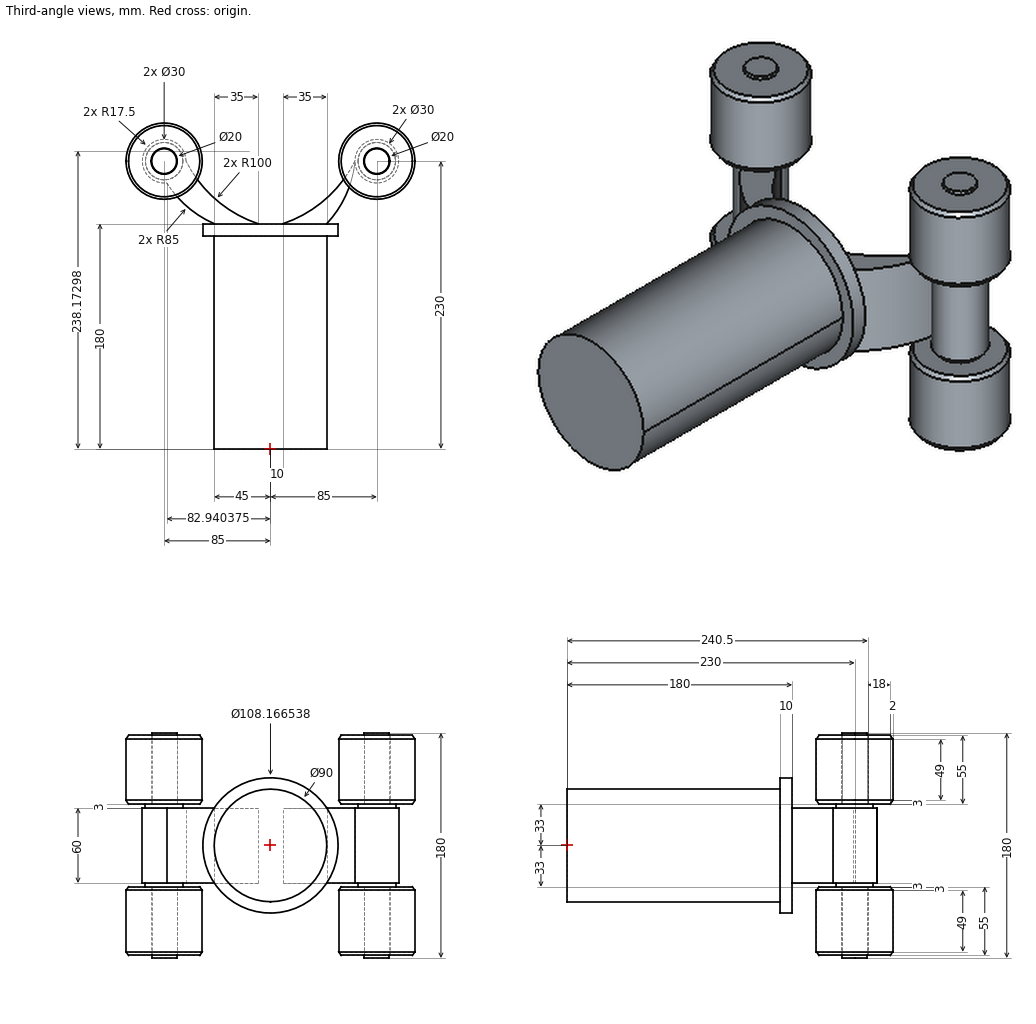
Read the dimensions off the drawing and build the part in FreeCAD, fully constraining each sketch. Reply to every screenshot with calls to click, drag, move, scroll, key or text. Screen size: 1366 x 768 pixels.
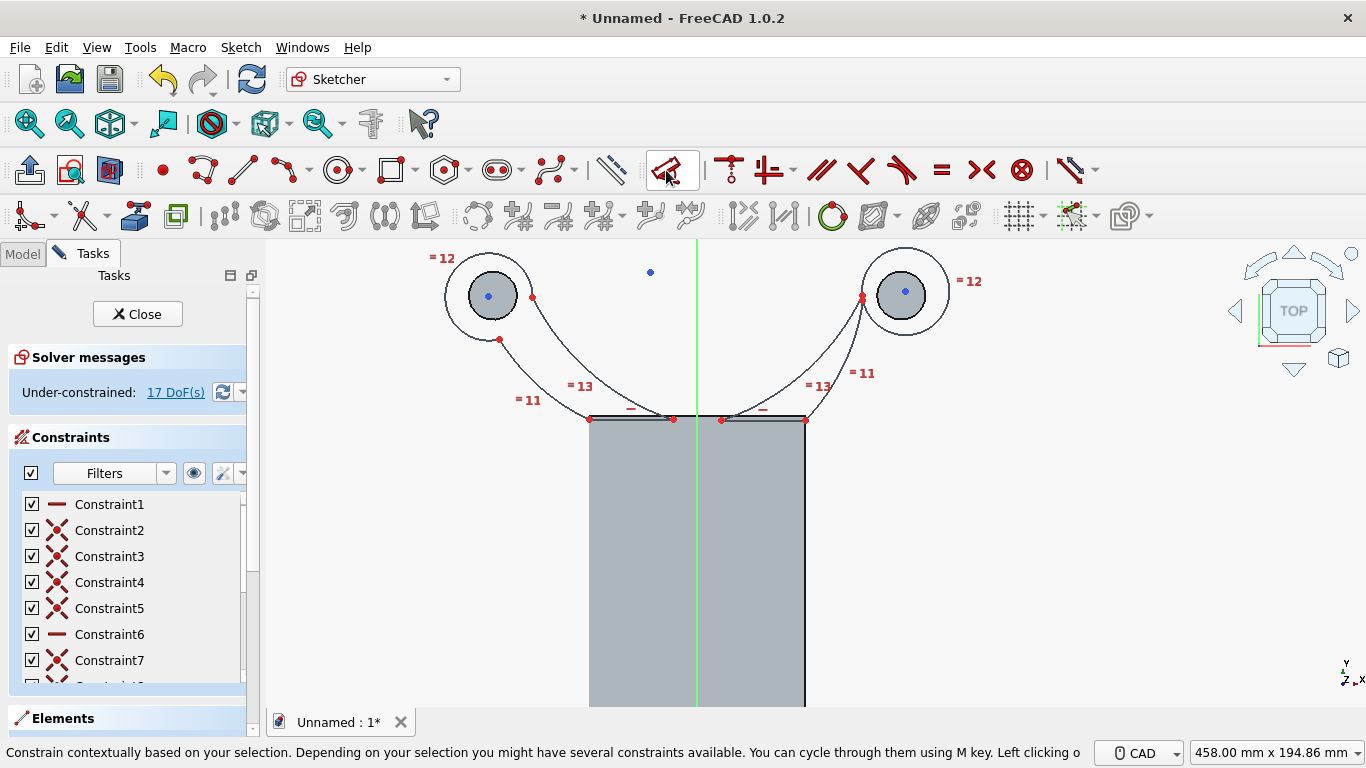
click(564, 345)
click(539, 366)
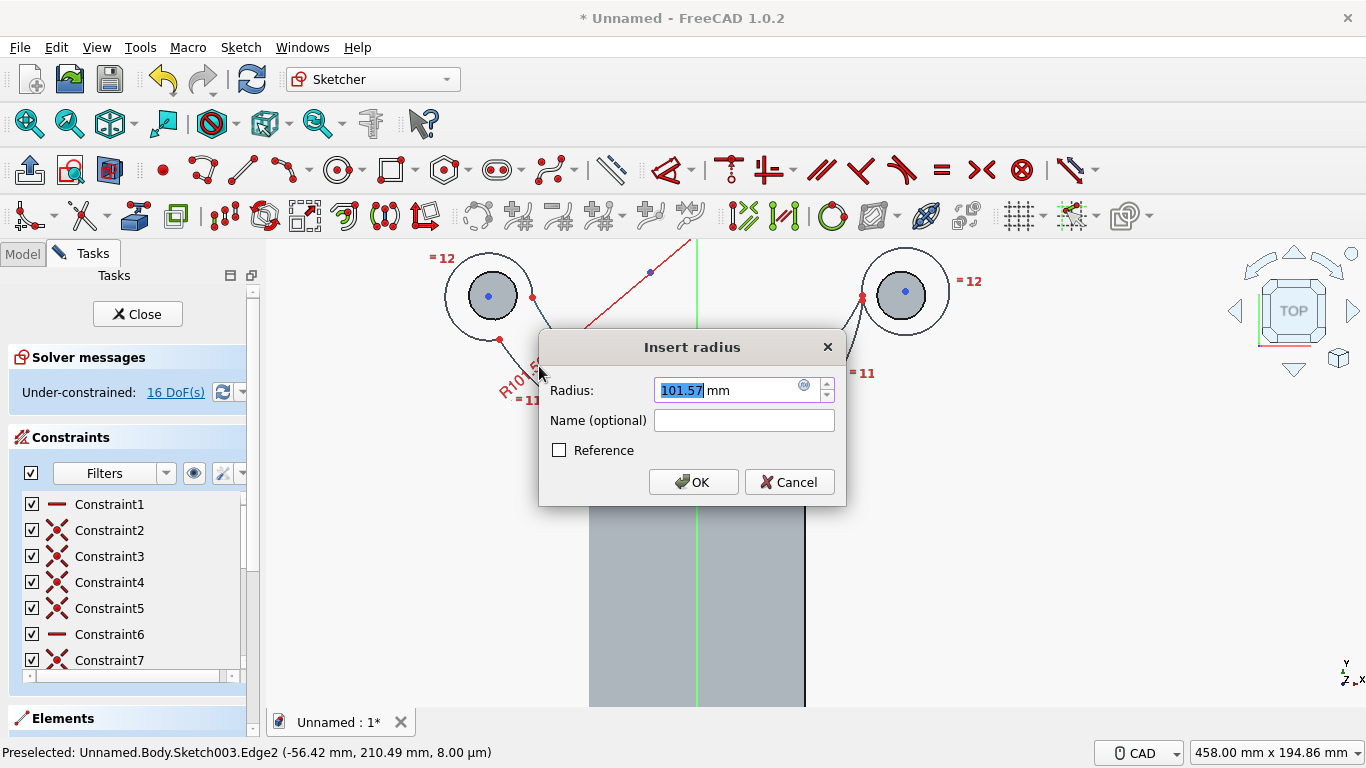
text(100)
key(Return)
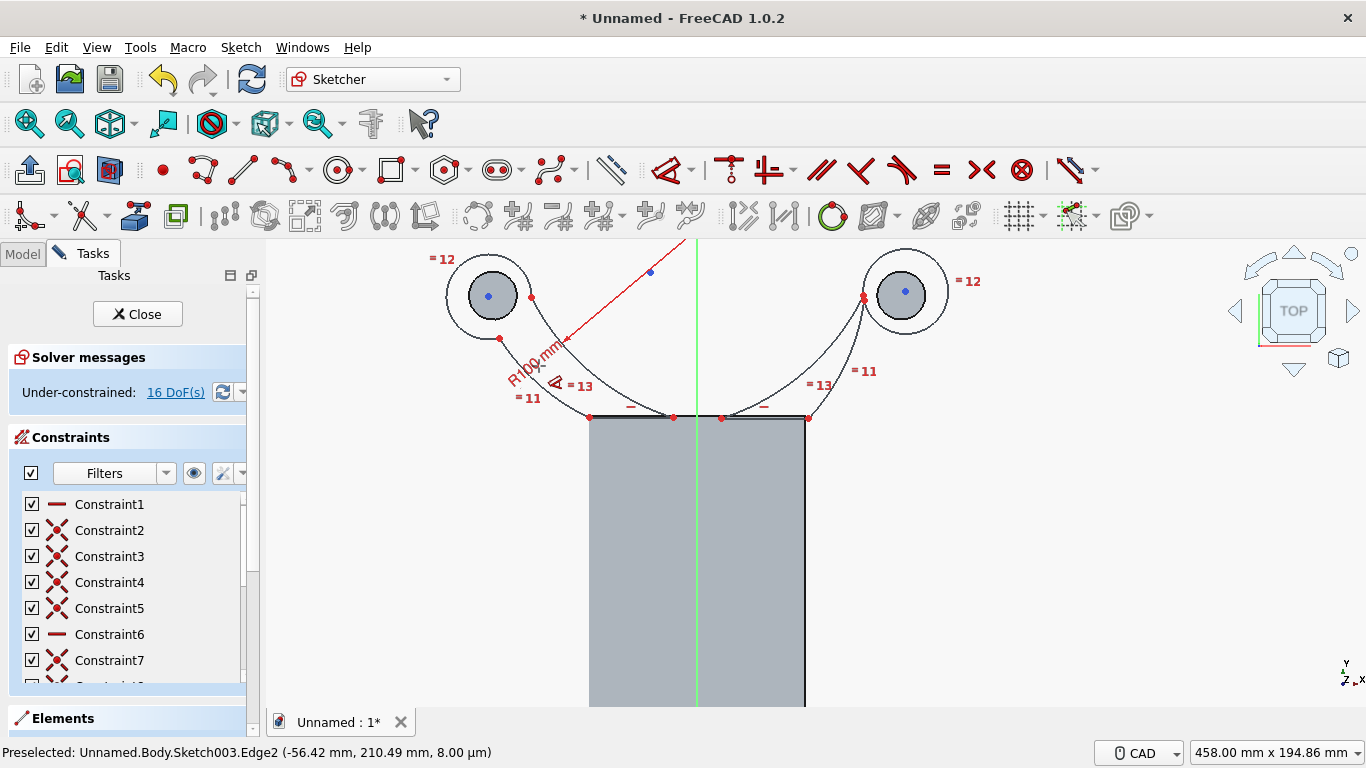
click(449, 311)
click(419, 322)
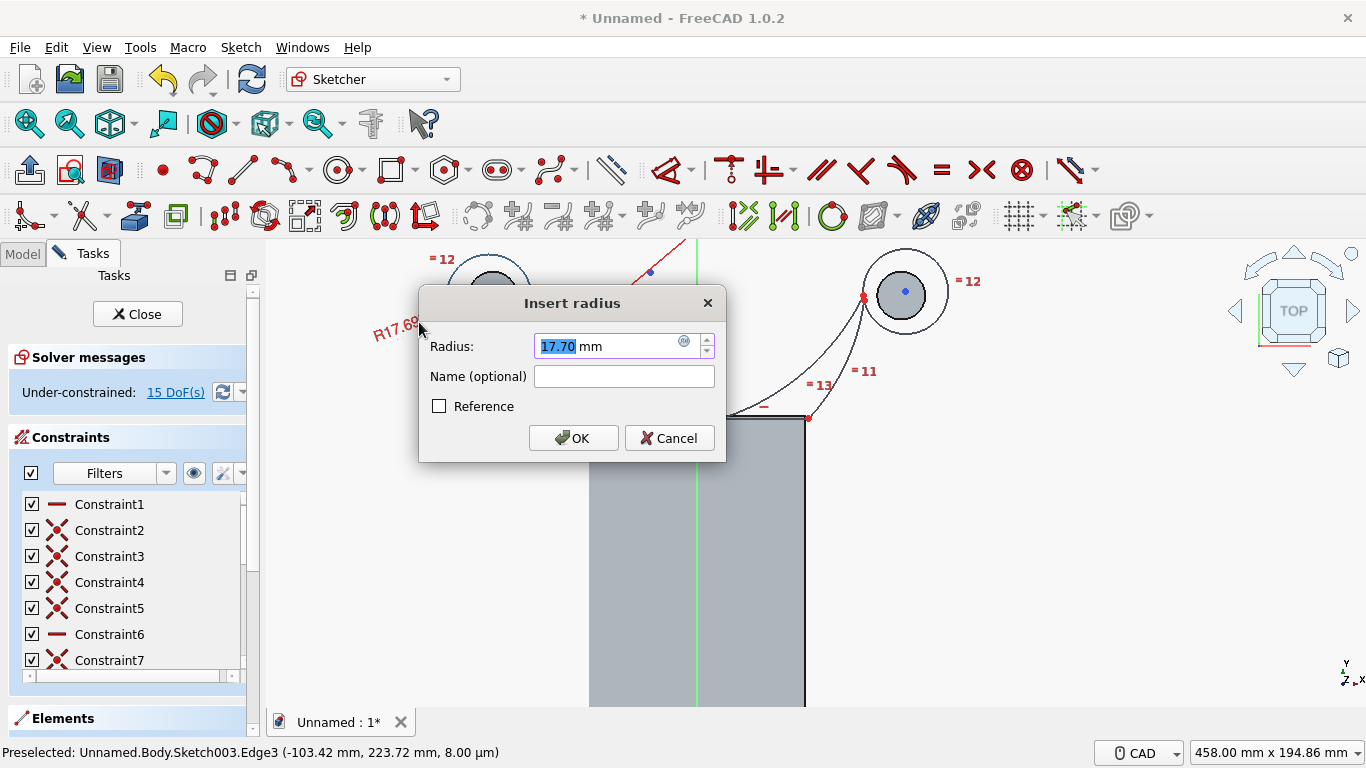
text(17.5)
key(Return)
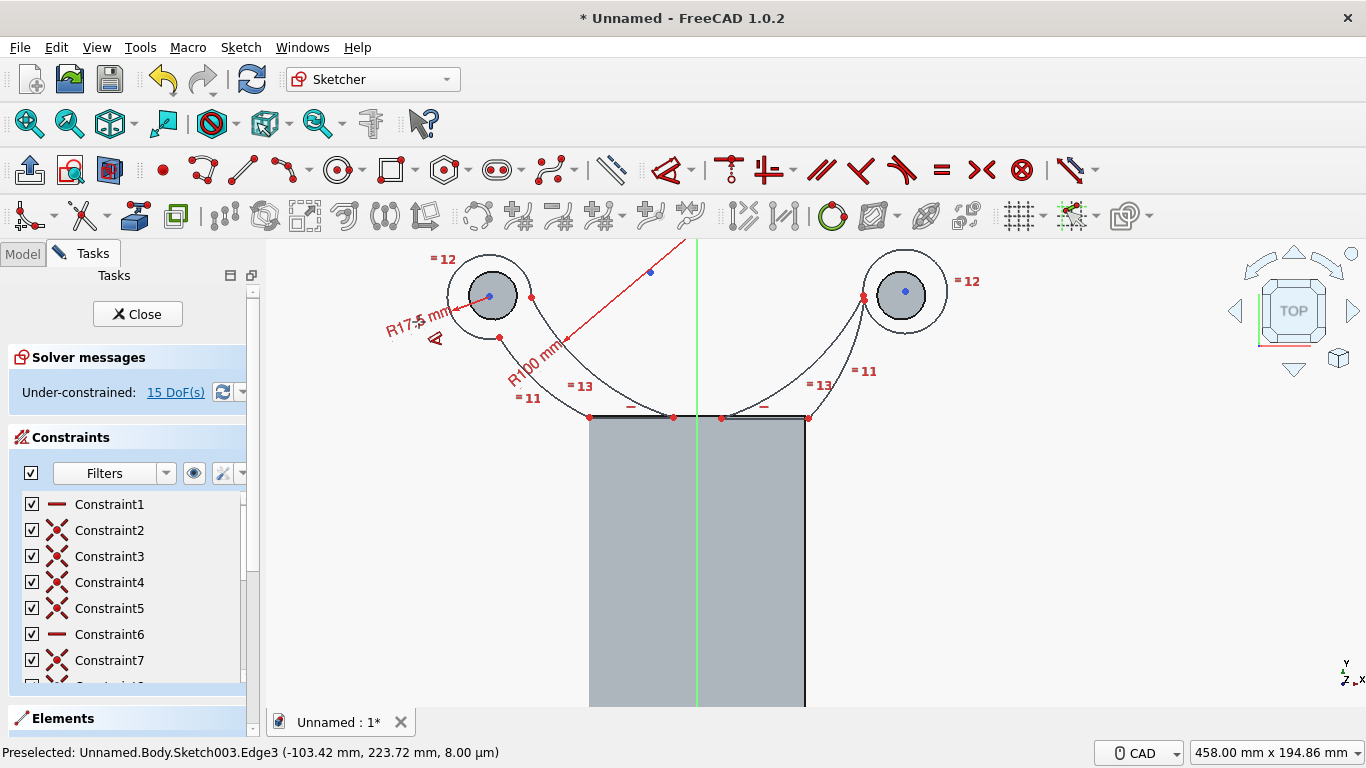
click(522, 367)
click(498, 388)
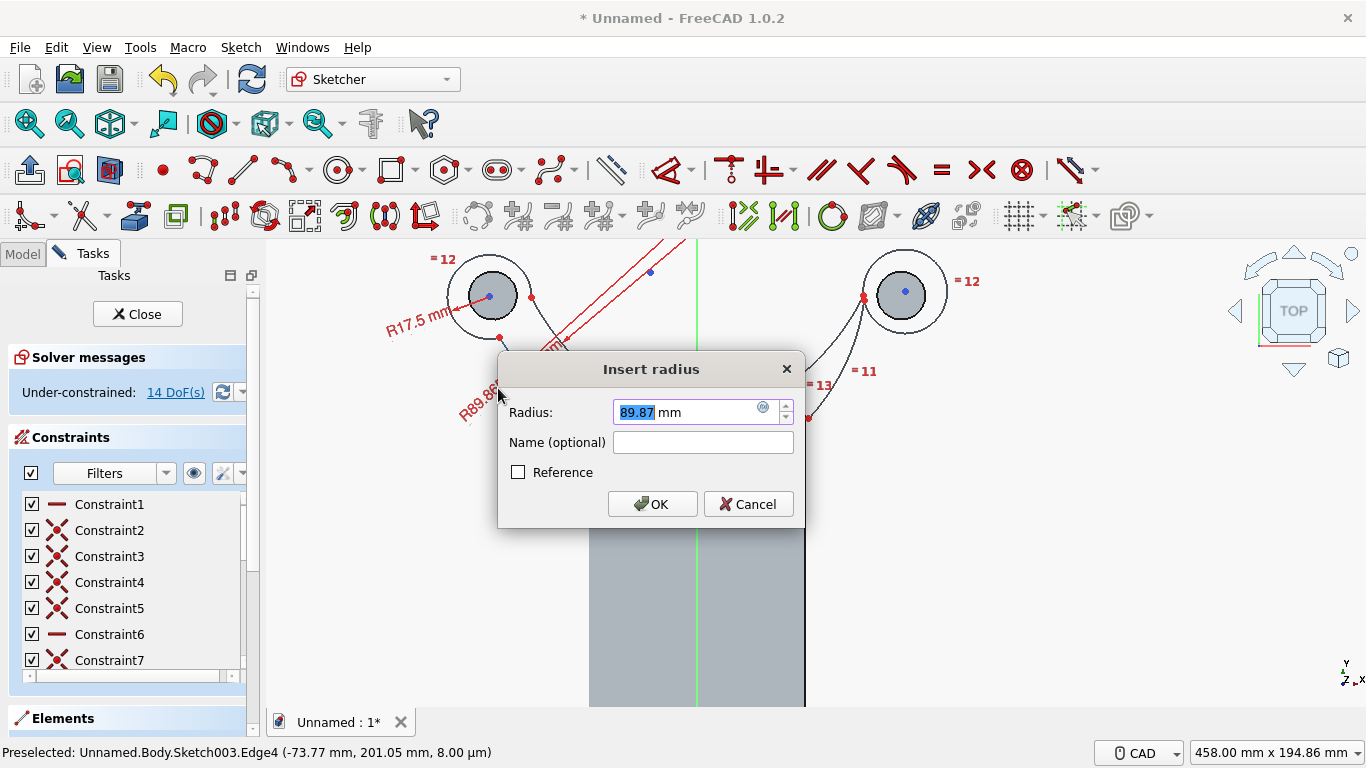
text(85)
key(Return)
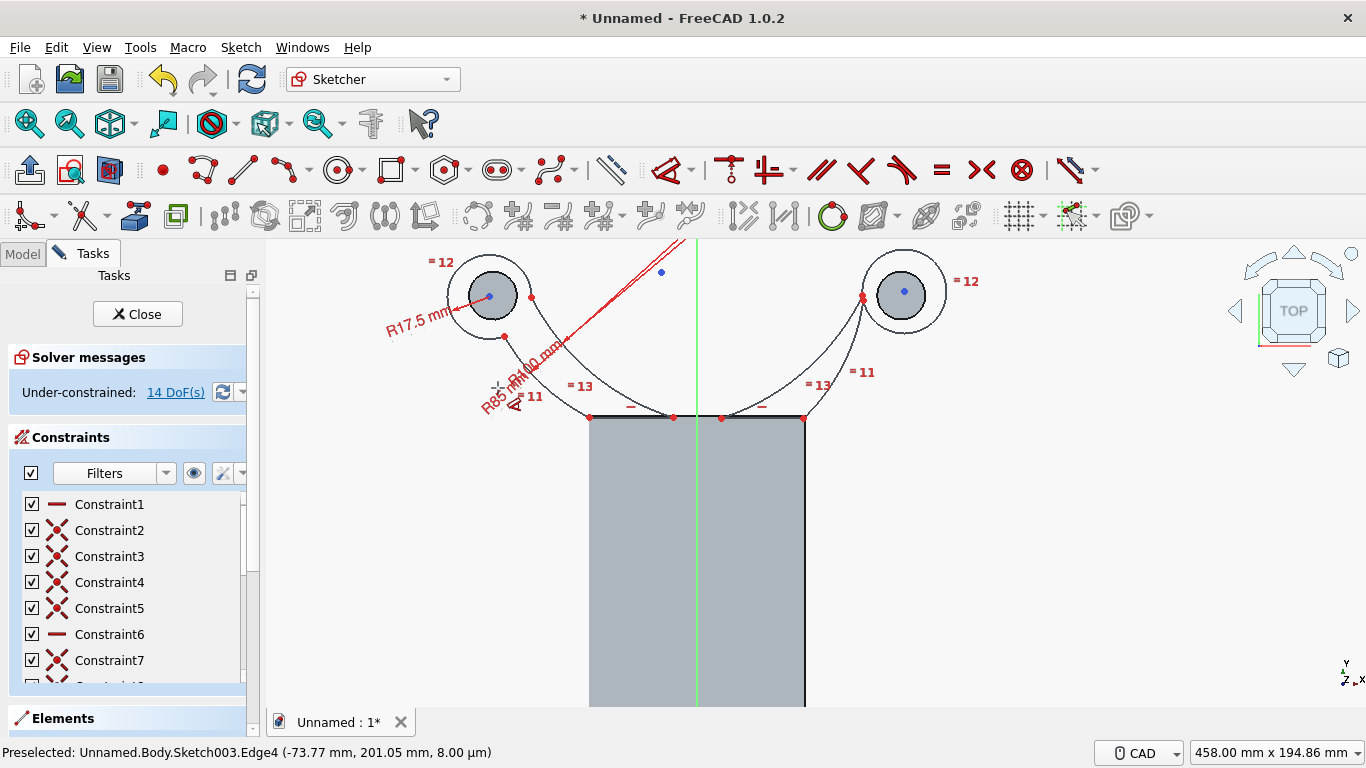
click(615, 418)
click(632, 384)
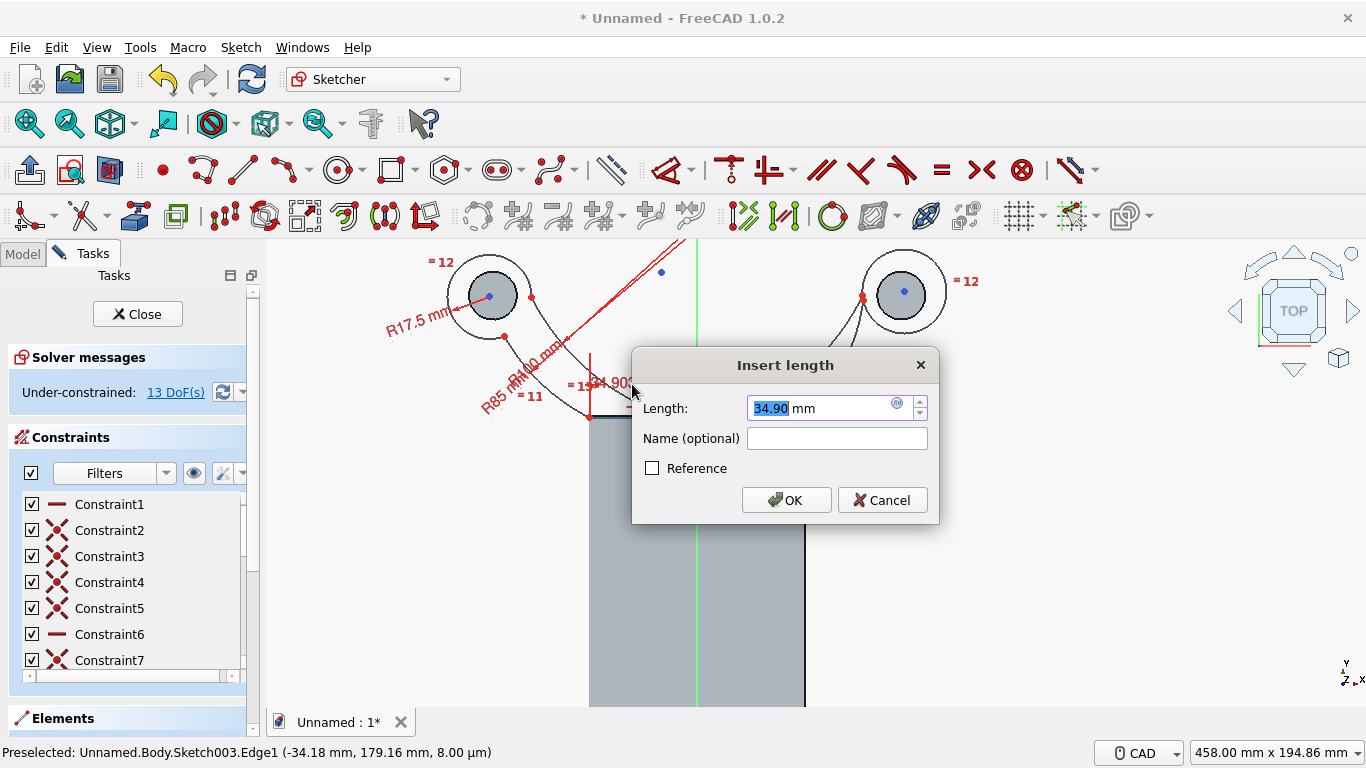
text(35)
key(Return)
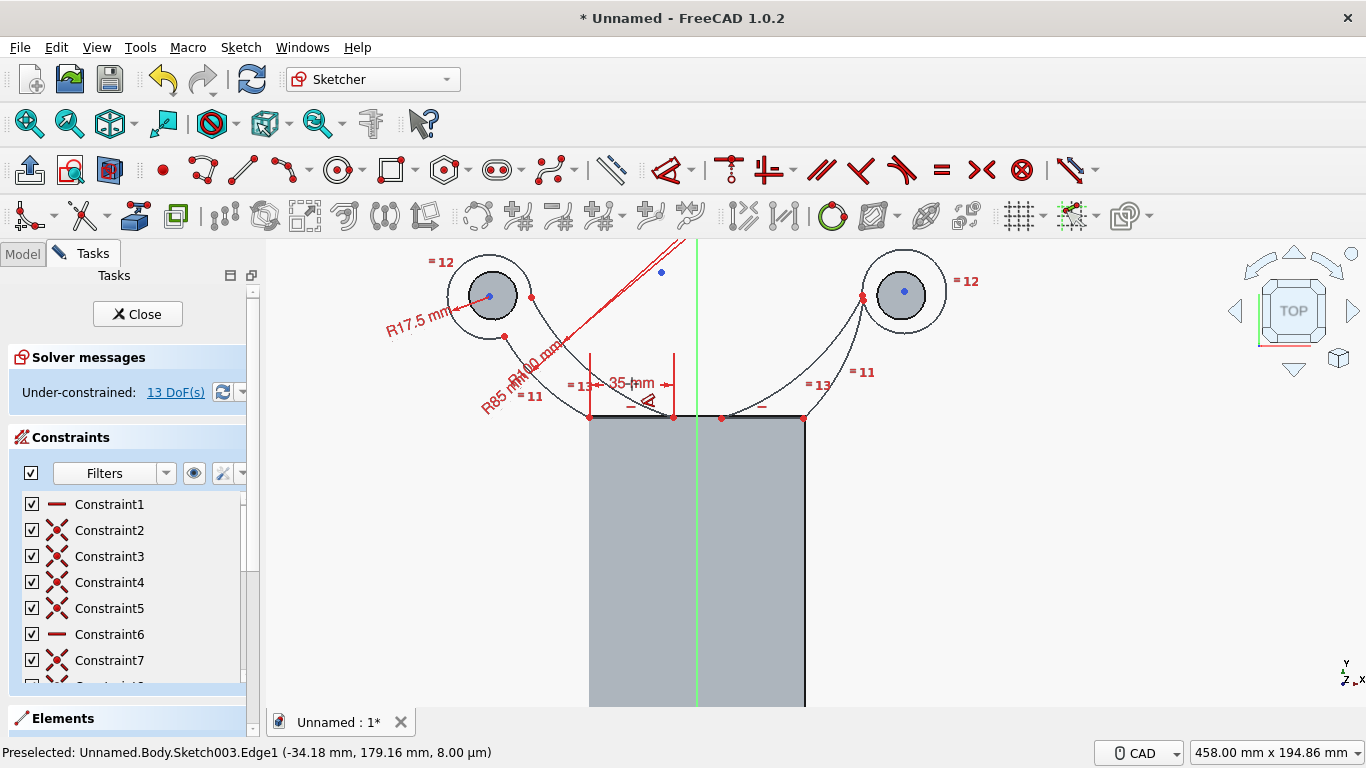
click(779, 418)
click(762, 384)